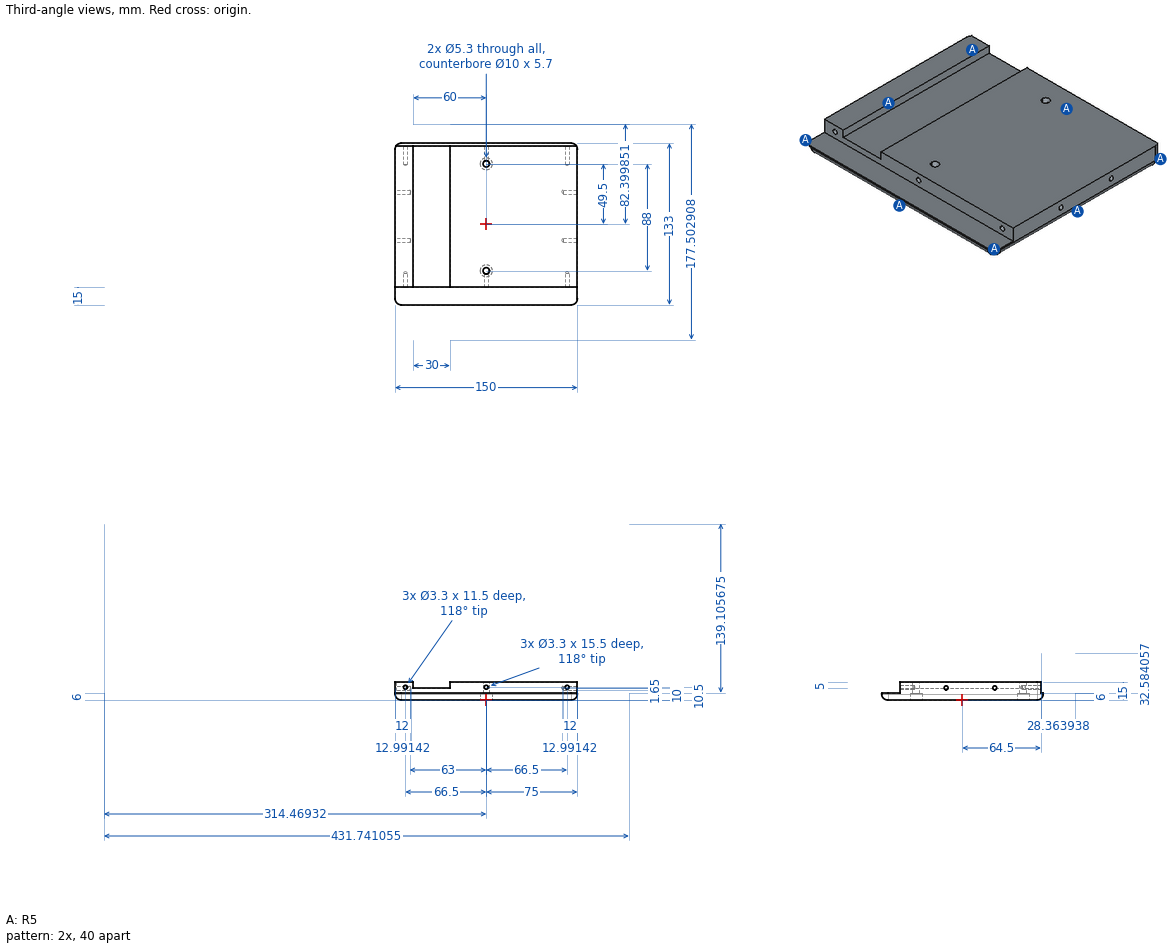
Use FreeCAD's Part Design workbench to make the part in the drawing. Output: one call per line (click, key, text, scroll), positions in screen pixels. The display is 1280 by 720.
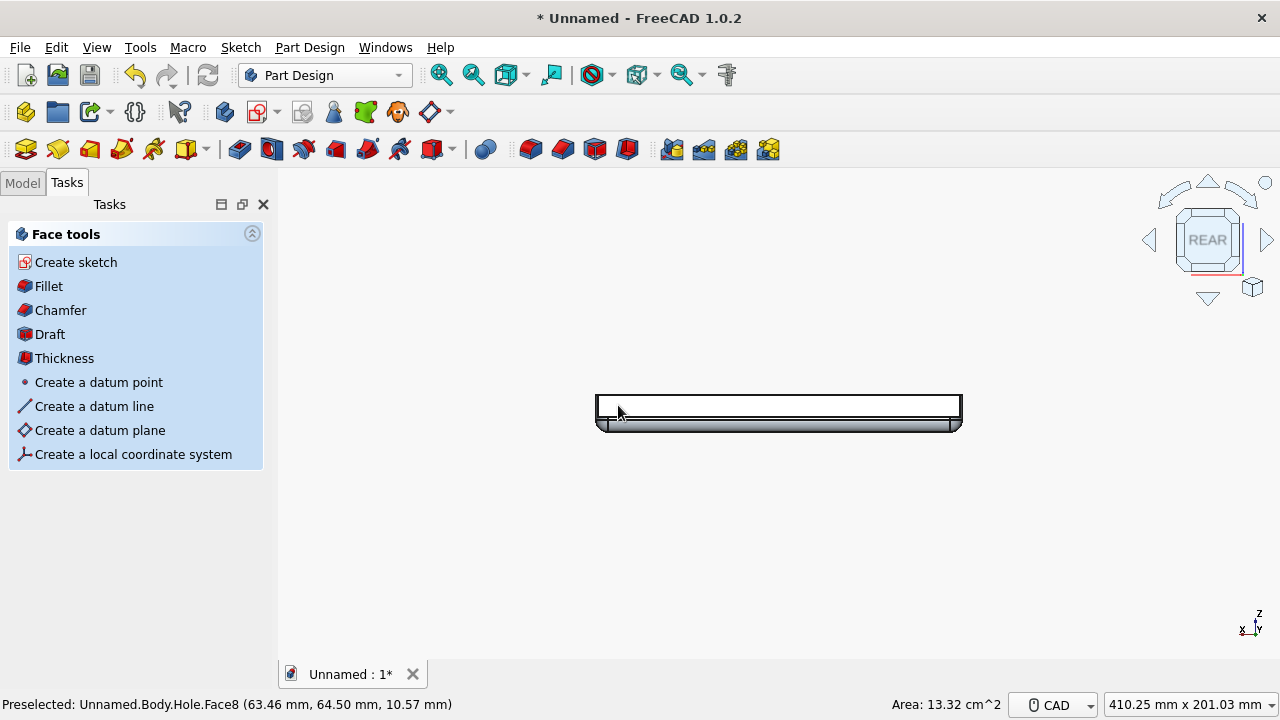
click(258, 112)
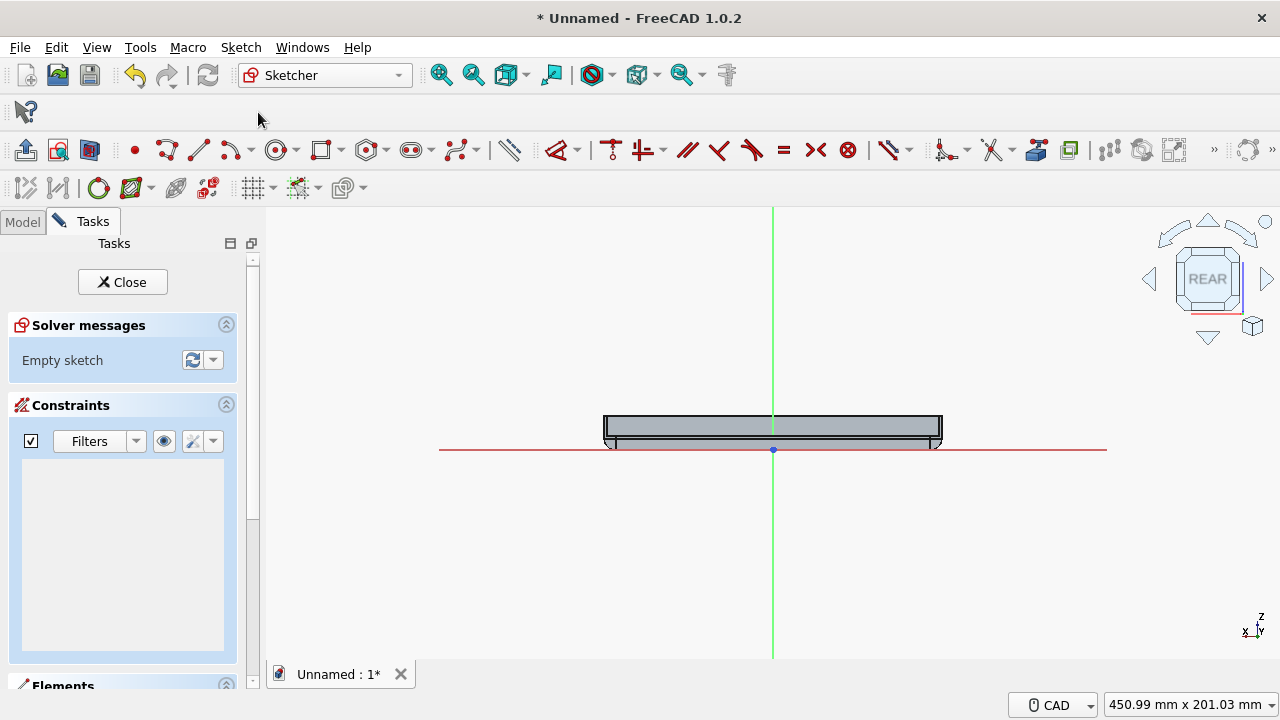
click(90, 150)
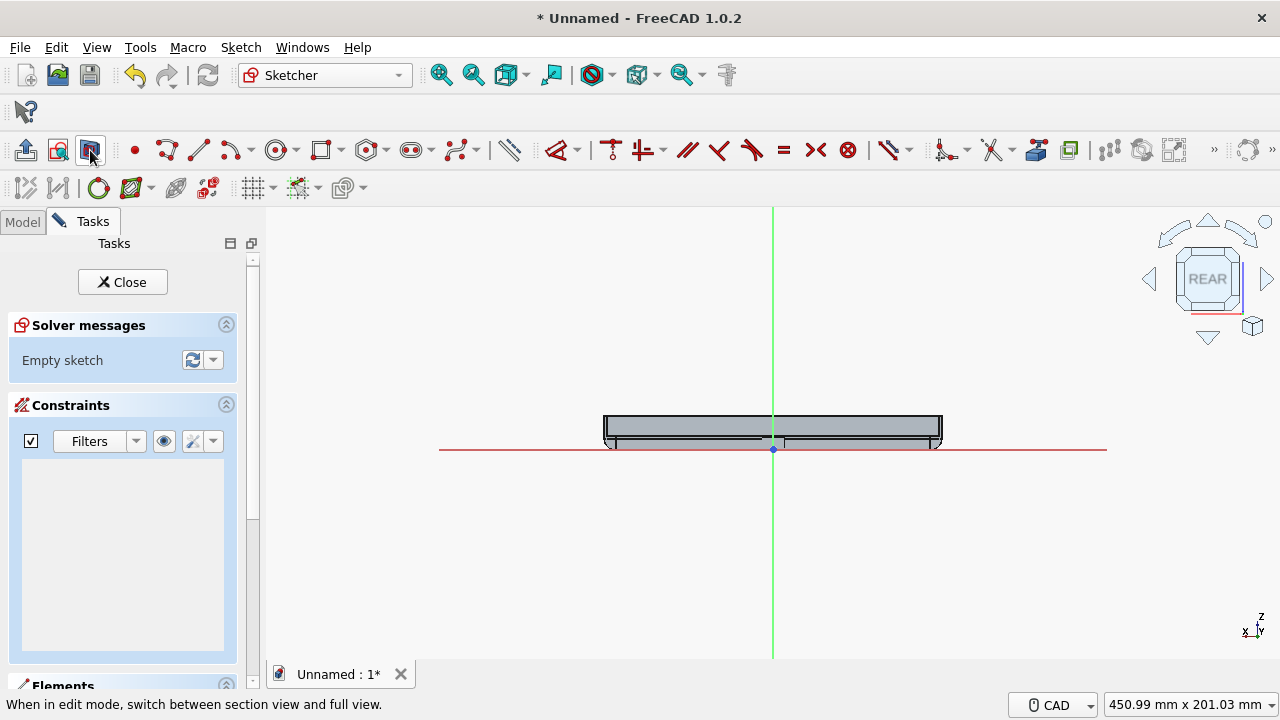
scroll(856, 440, up, 3)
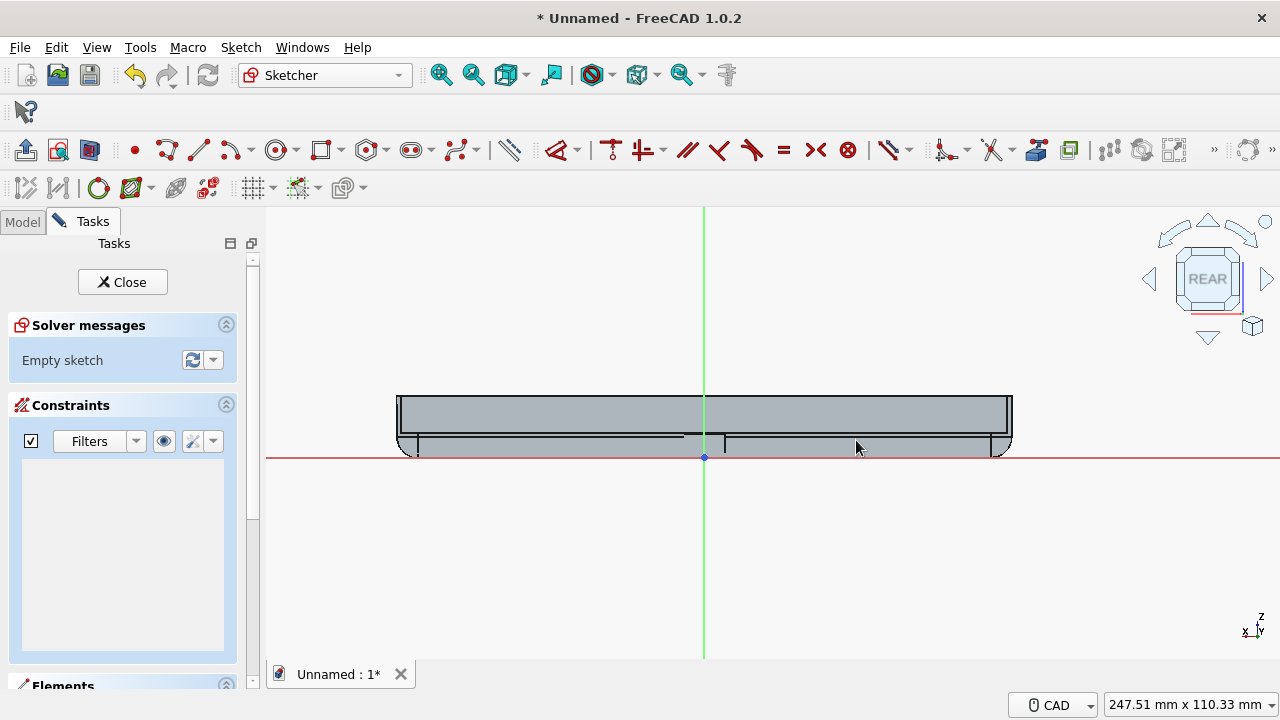
click(276, 150)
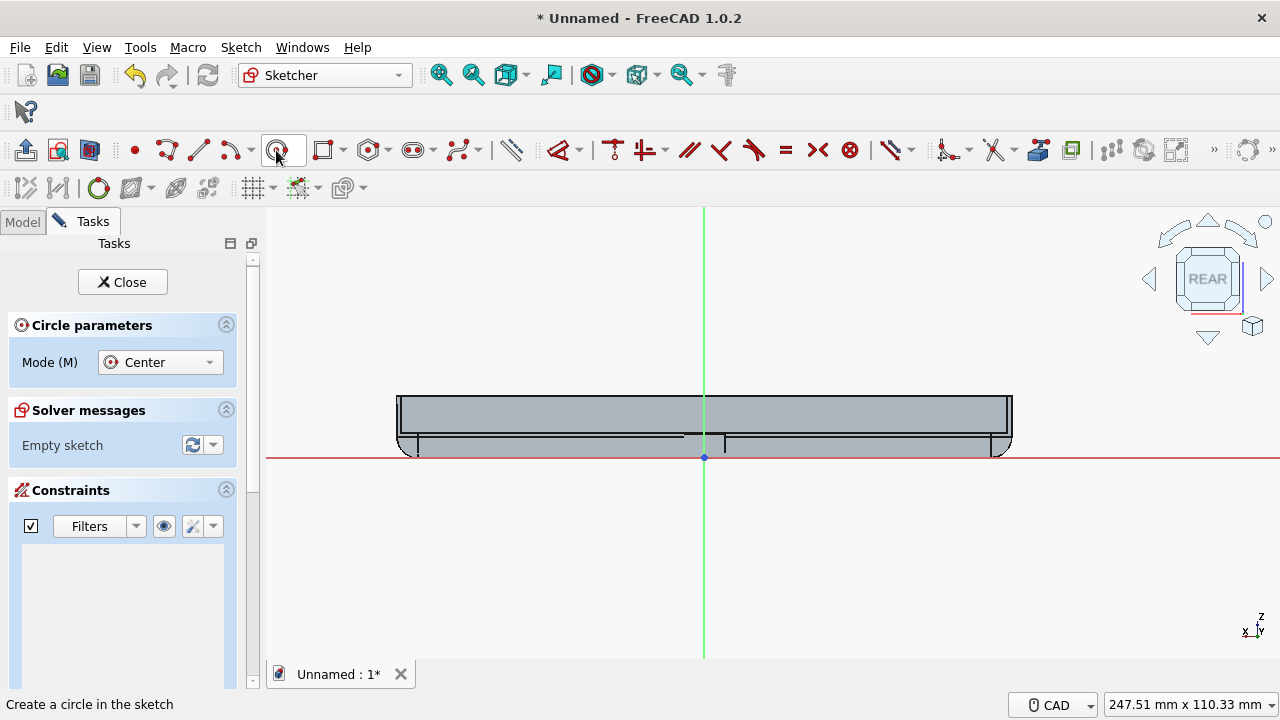
scroll(704, 415, up, 7)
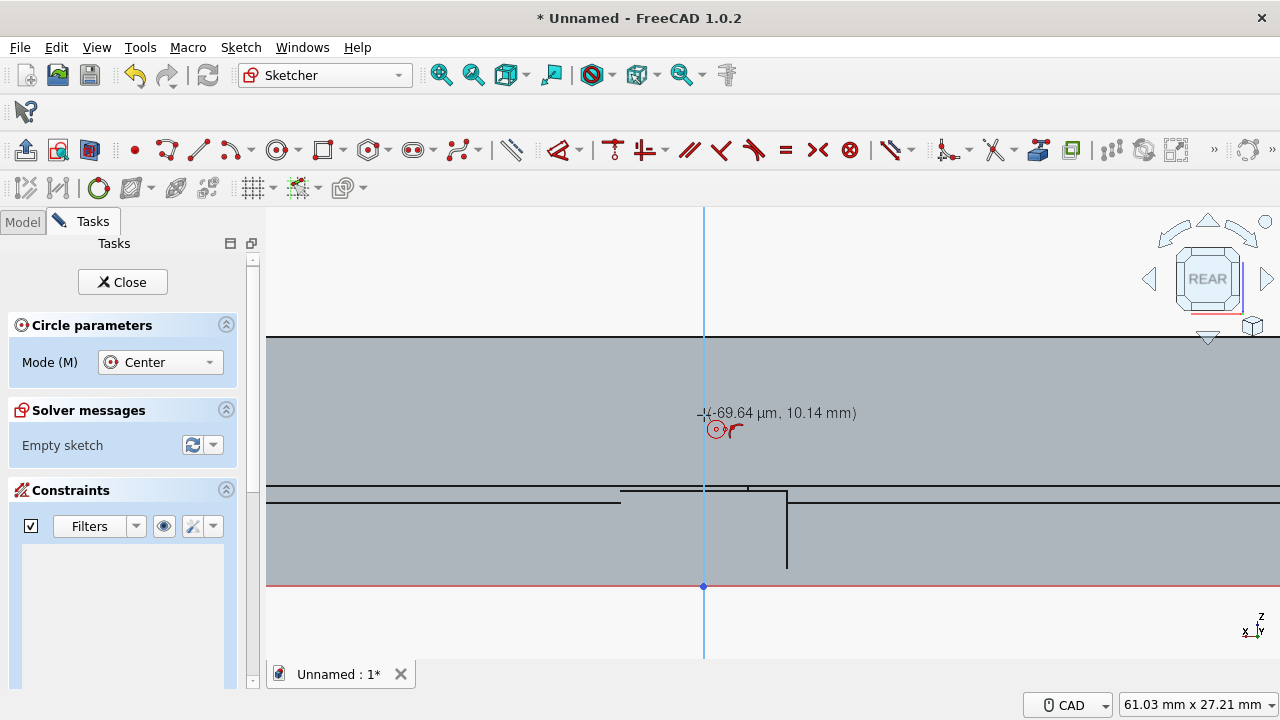
scroll(705, 416, down, 7)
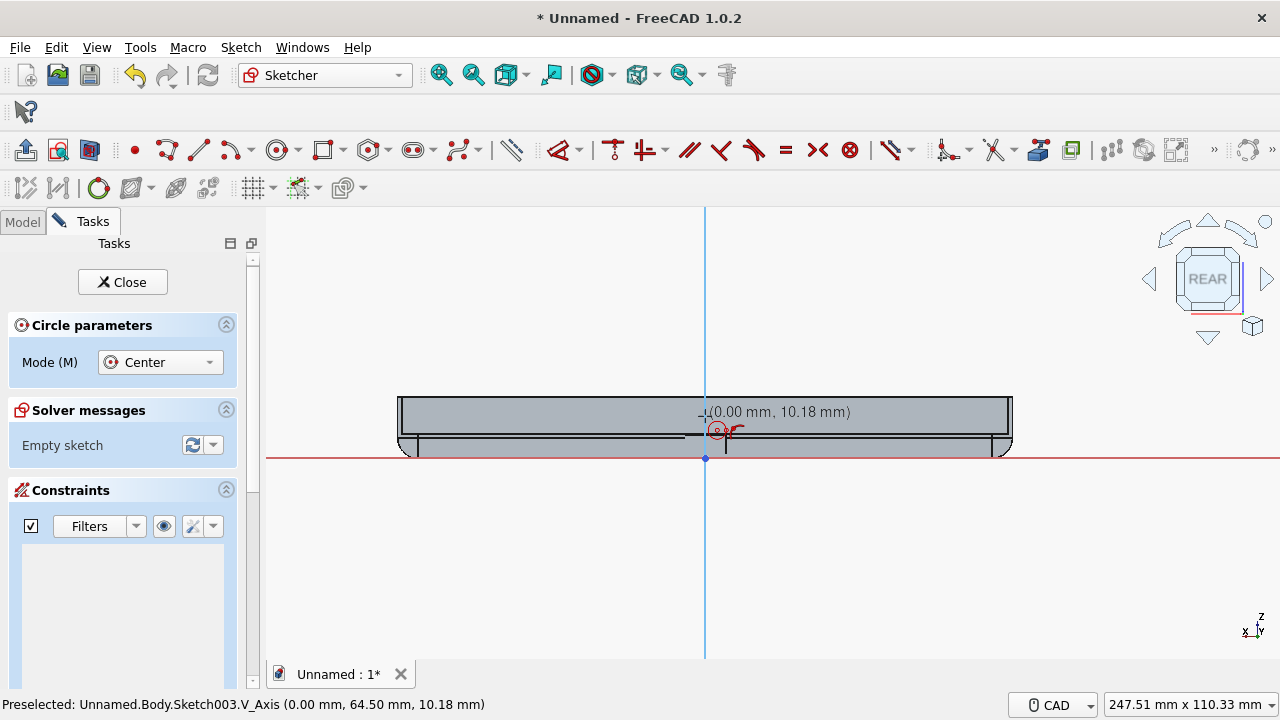
click(705, 415)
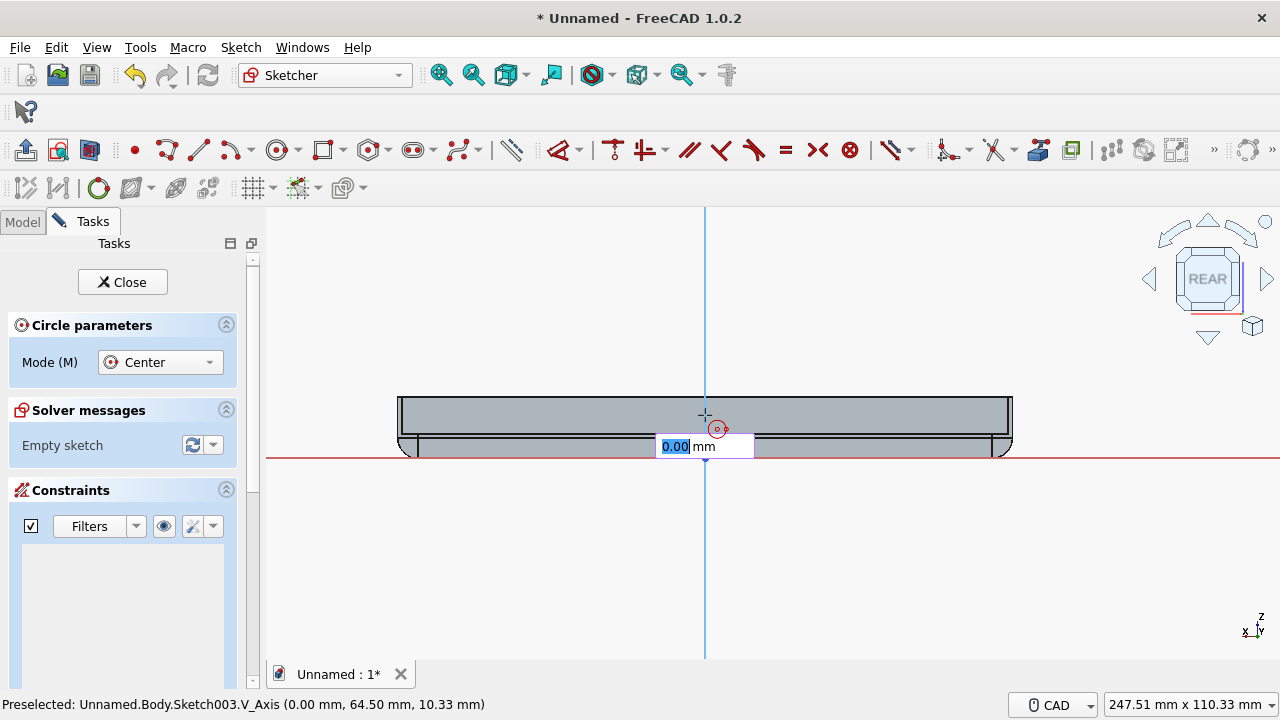
scroll(711, 413, up, 5)
move(711, 412)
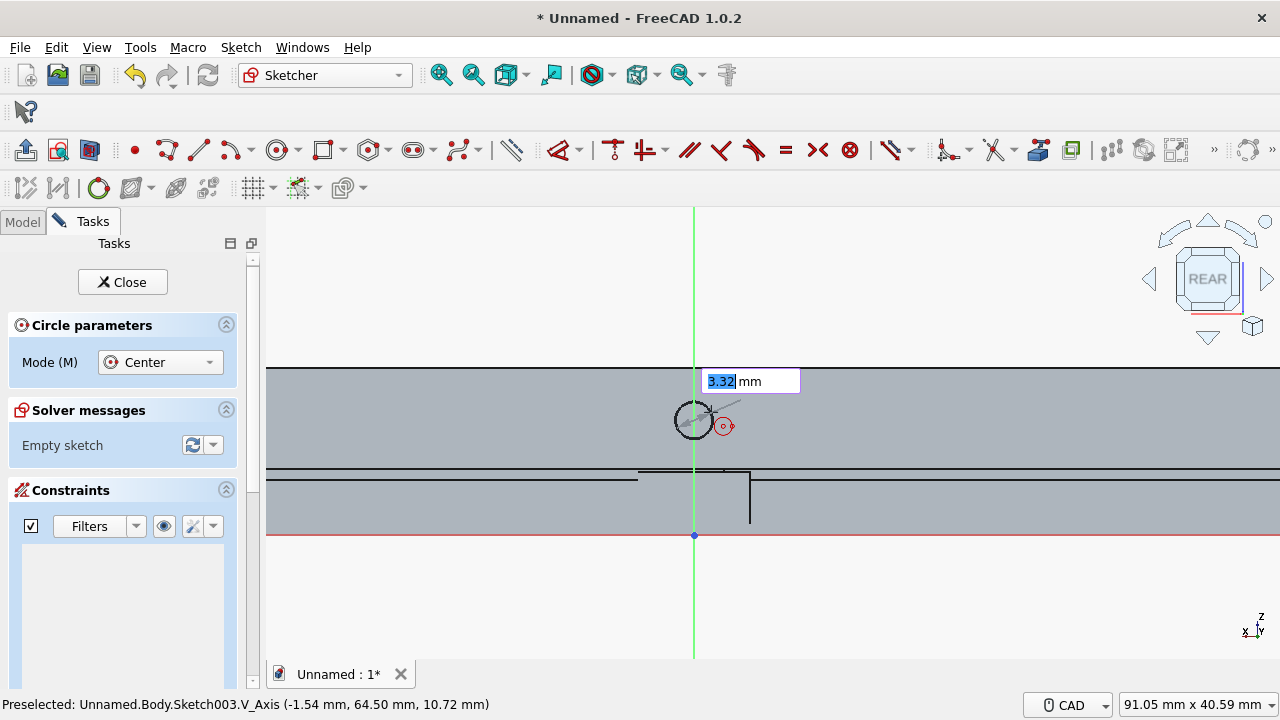
text(3.3)
key(Return)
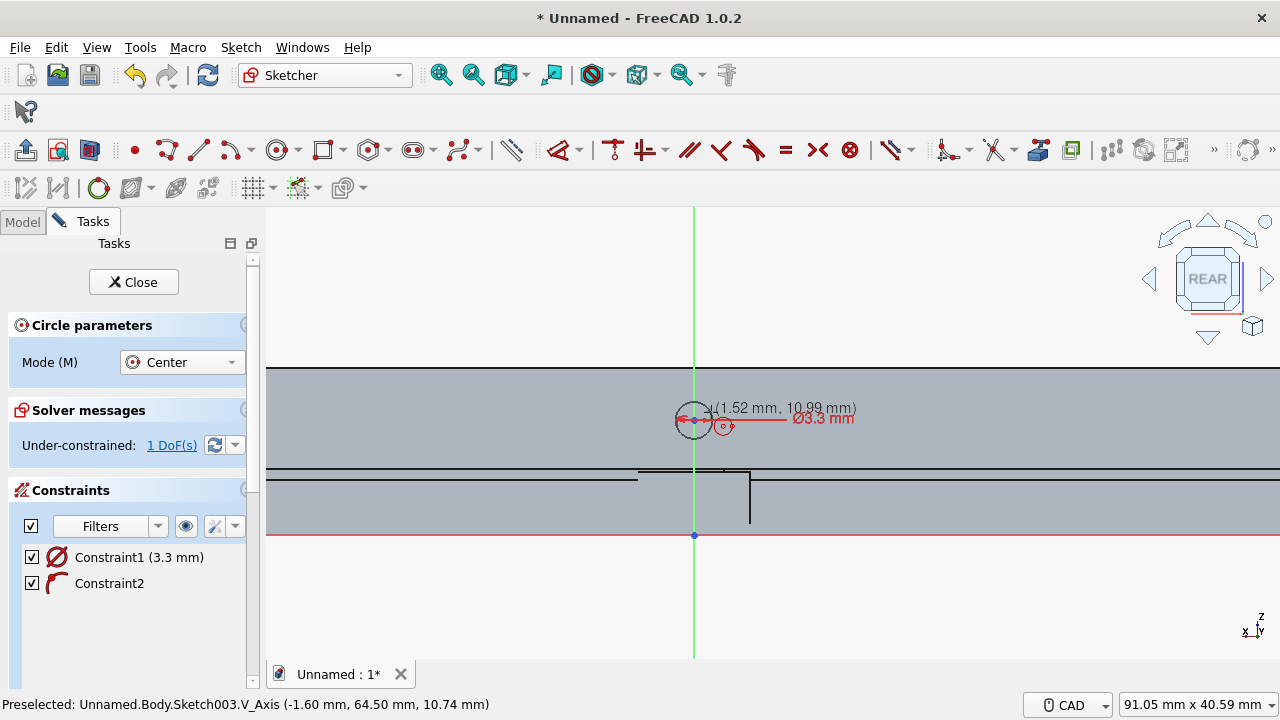
scroll(711, 413, down, 5)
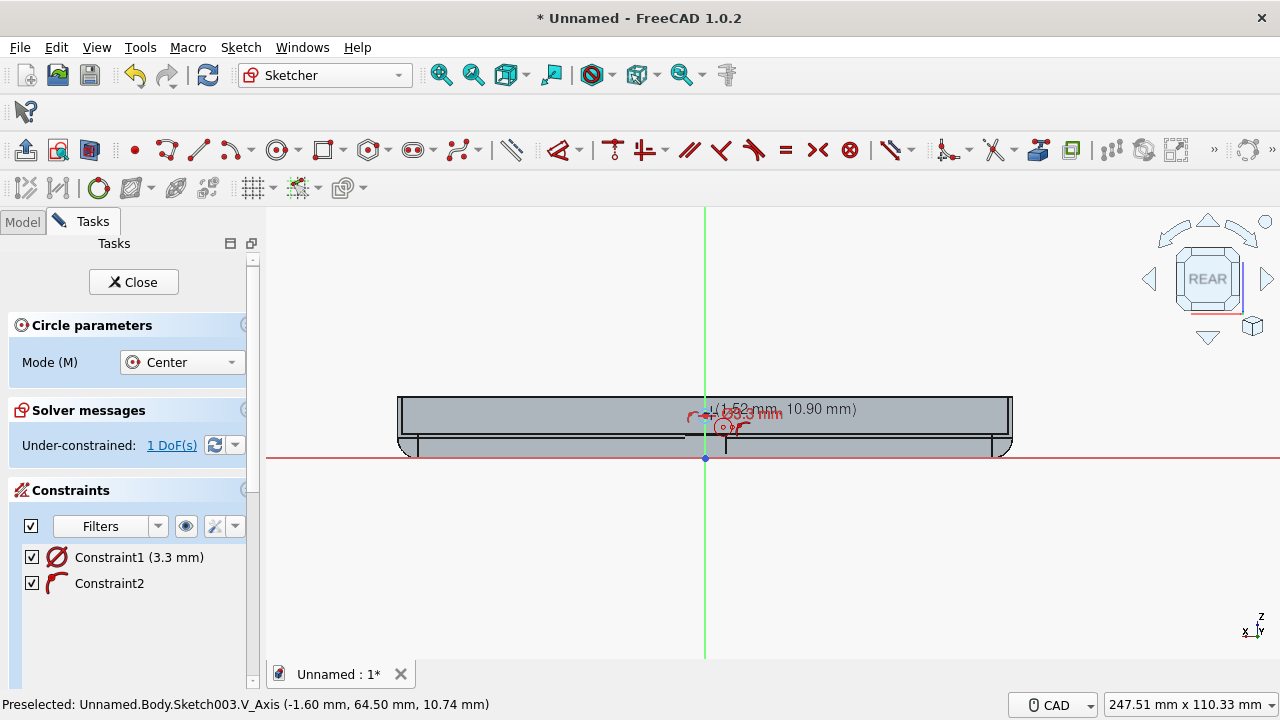
scroll(433, 415, up, 7)